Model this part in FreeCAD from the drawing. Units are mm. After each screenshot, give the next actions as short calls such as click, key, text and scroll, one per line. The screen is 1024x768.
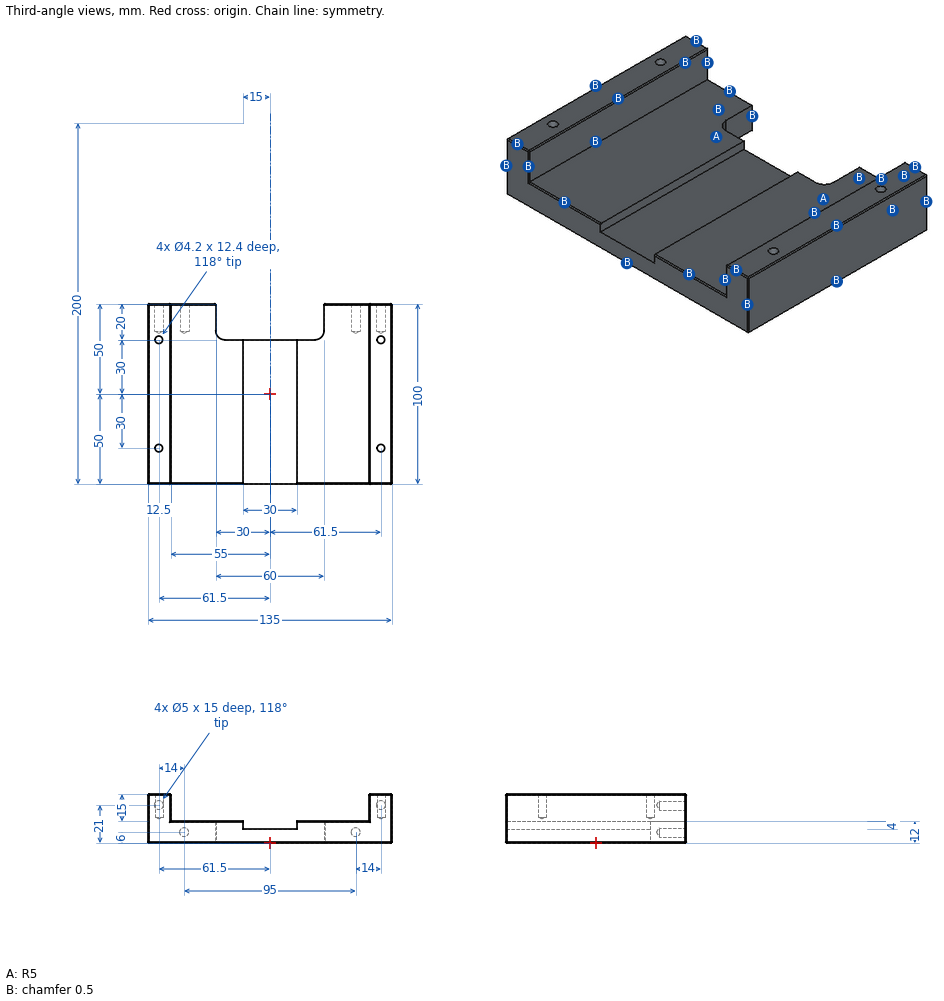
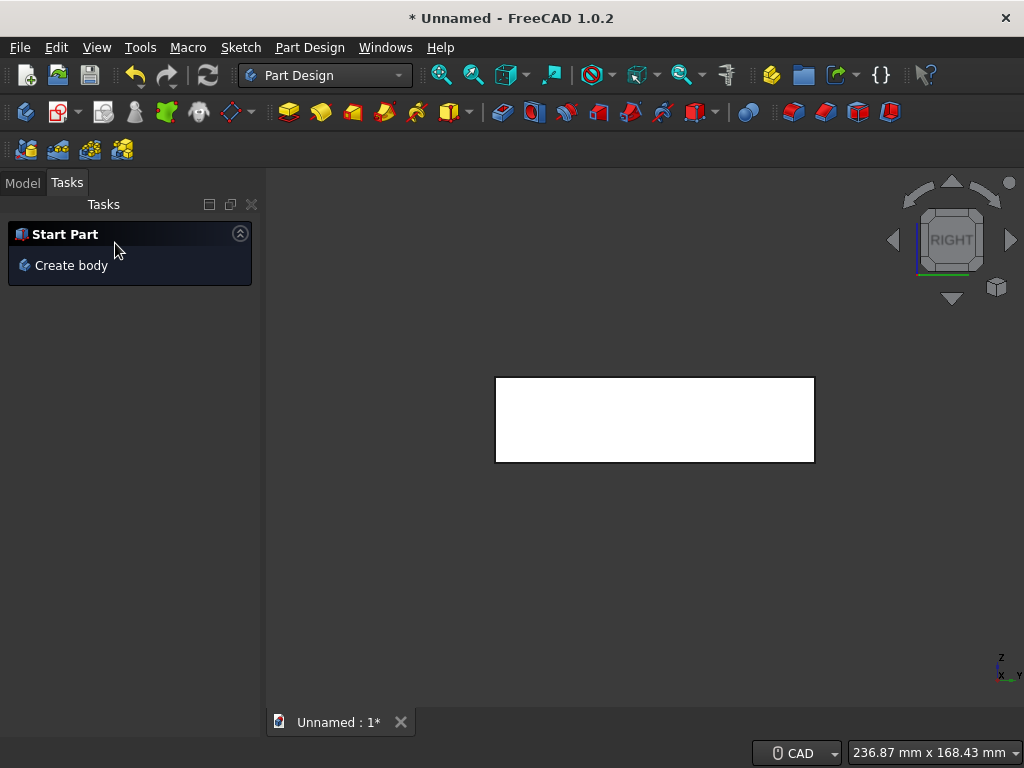
click(442, 76)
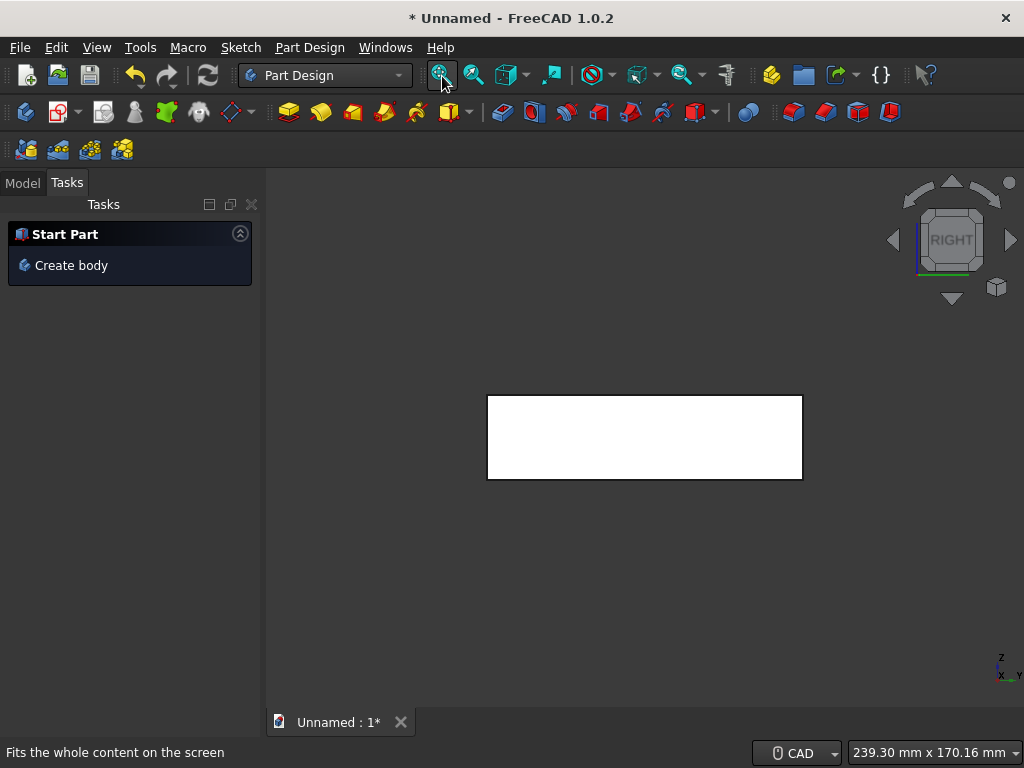
key(5)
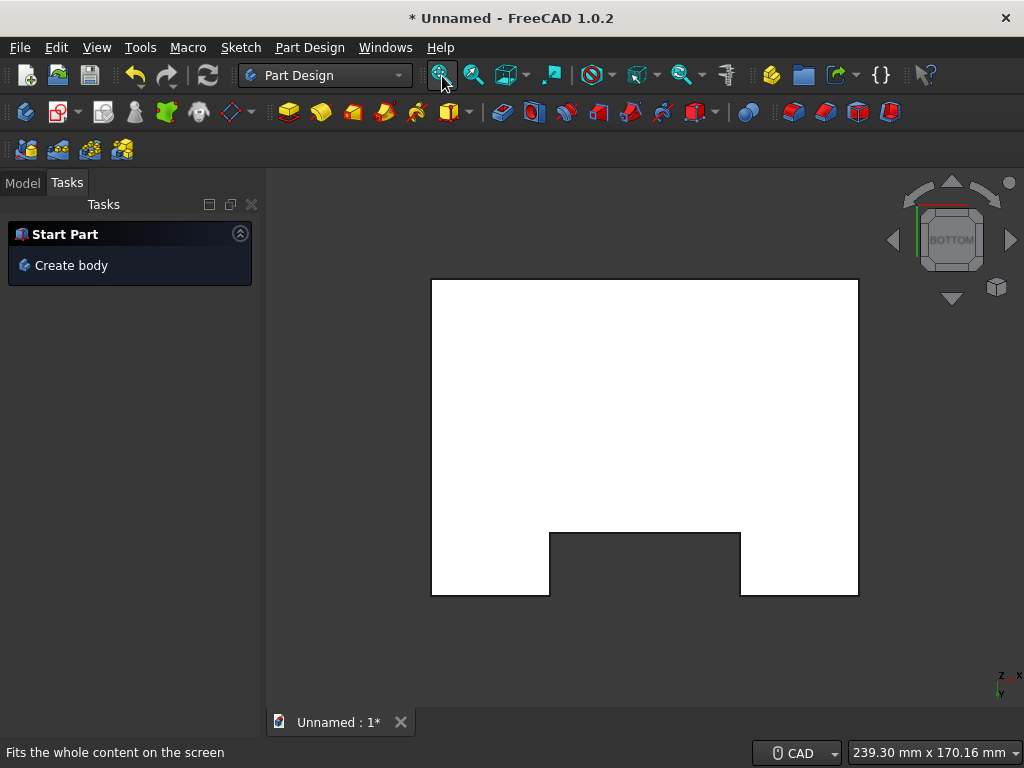
key(4)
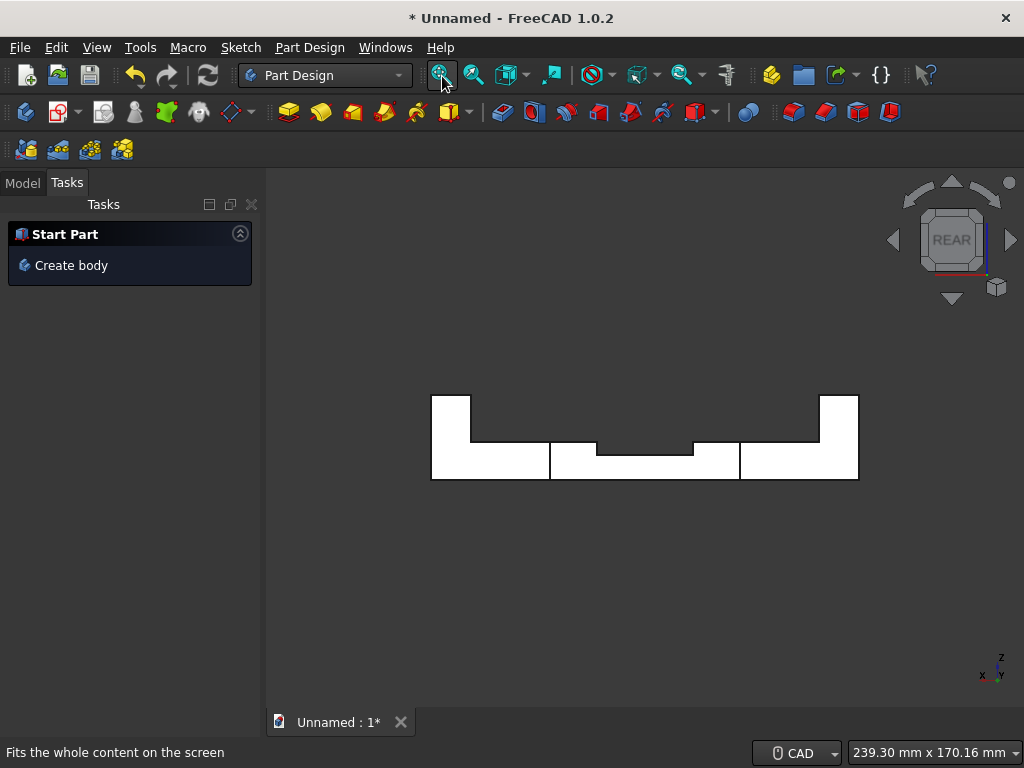
key(6)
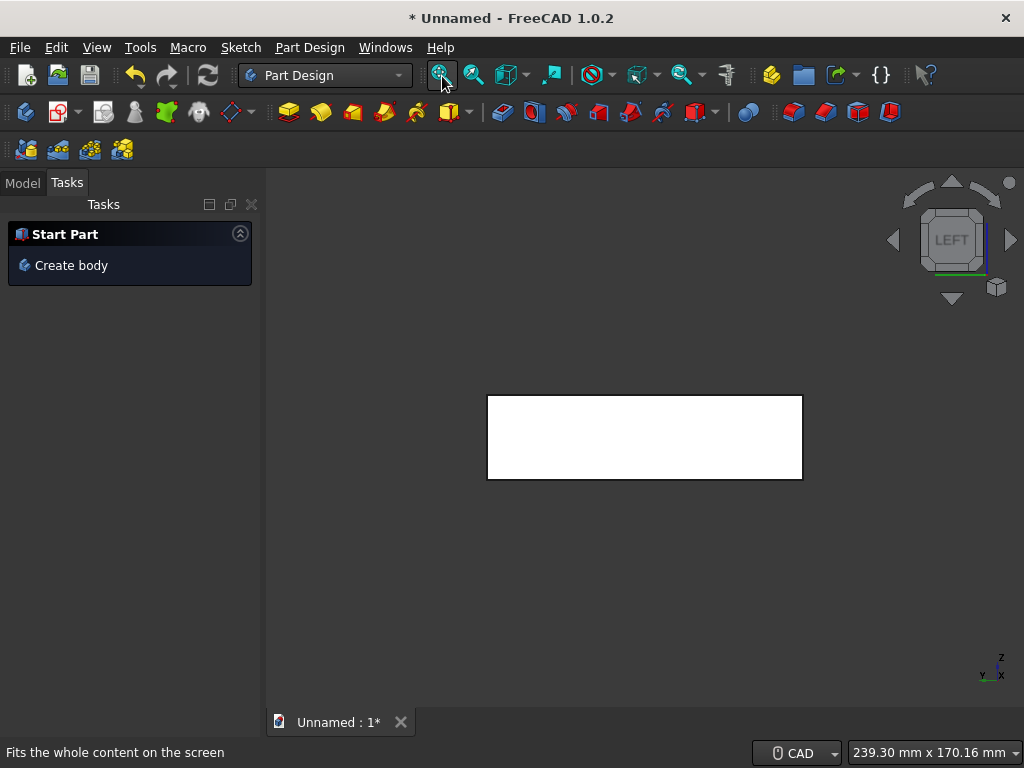
click(442, 76)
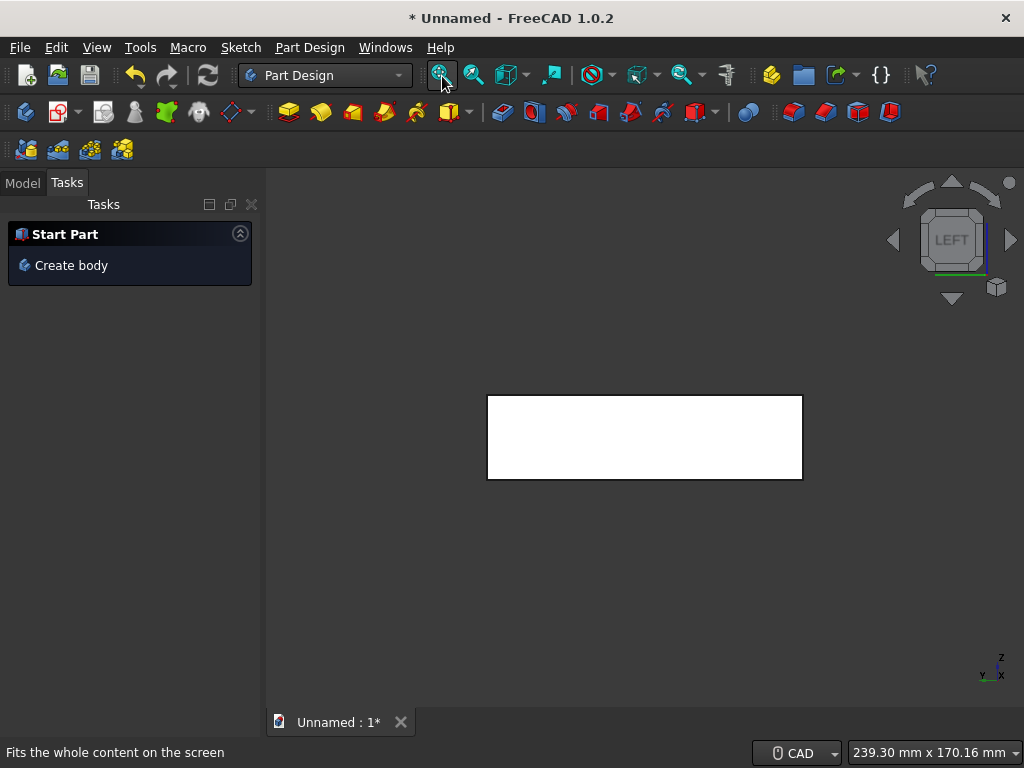
key(v)
key(3)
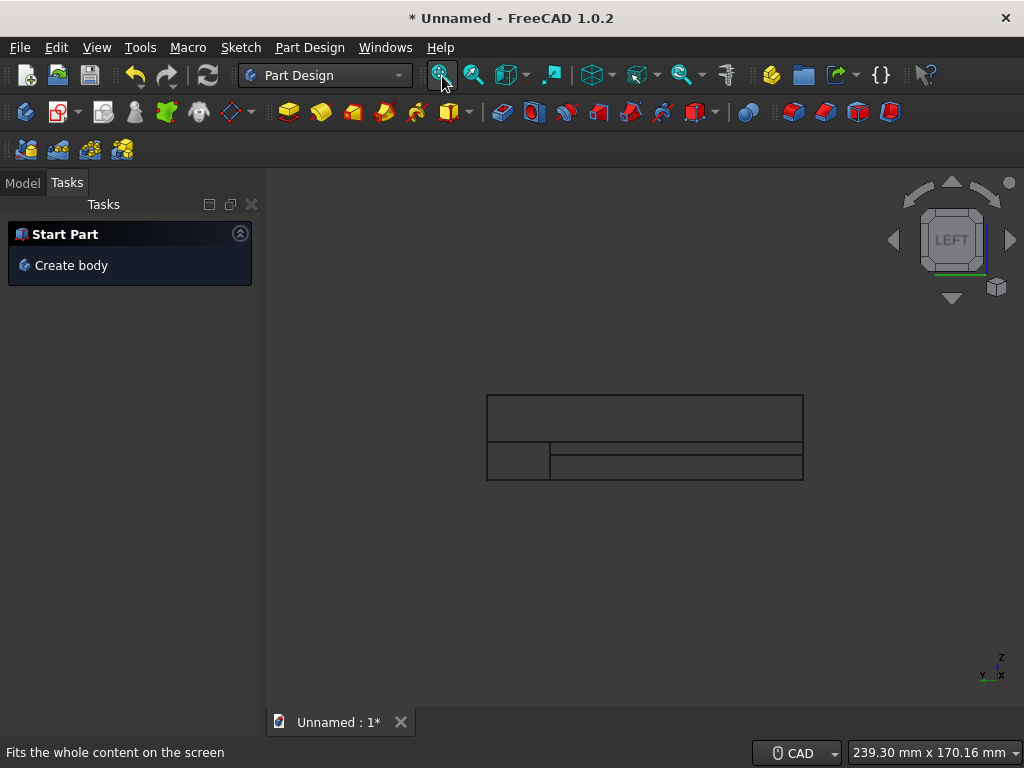
key(0)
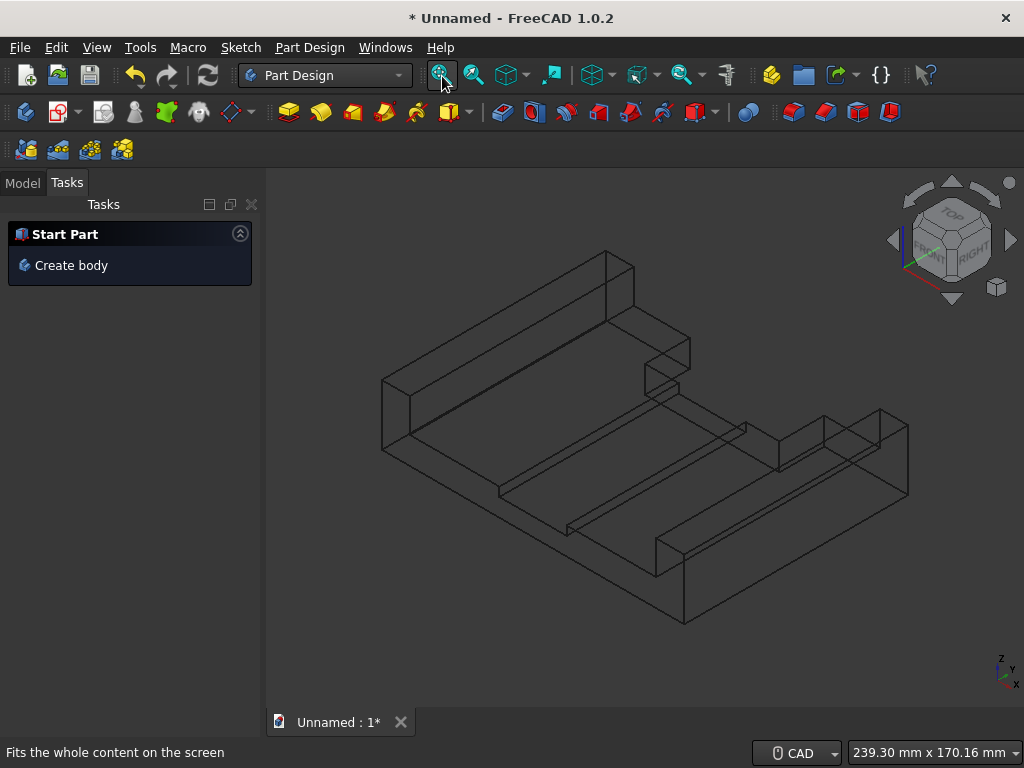
click(779, 456)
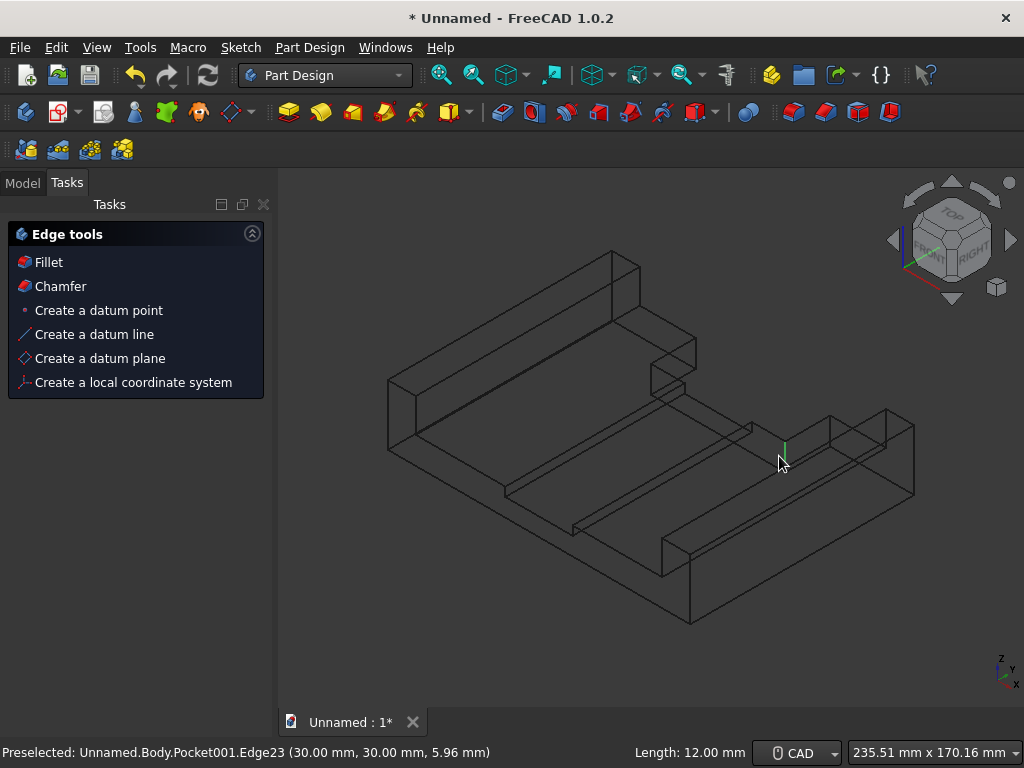
click(651, 378, ctrl)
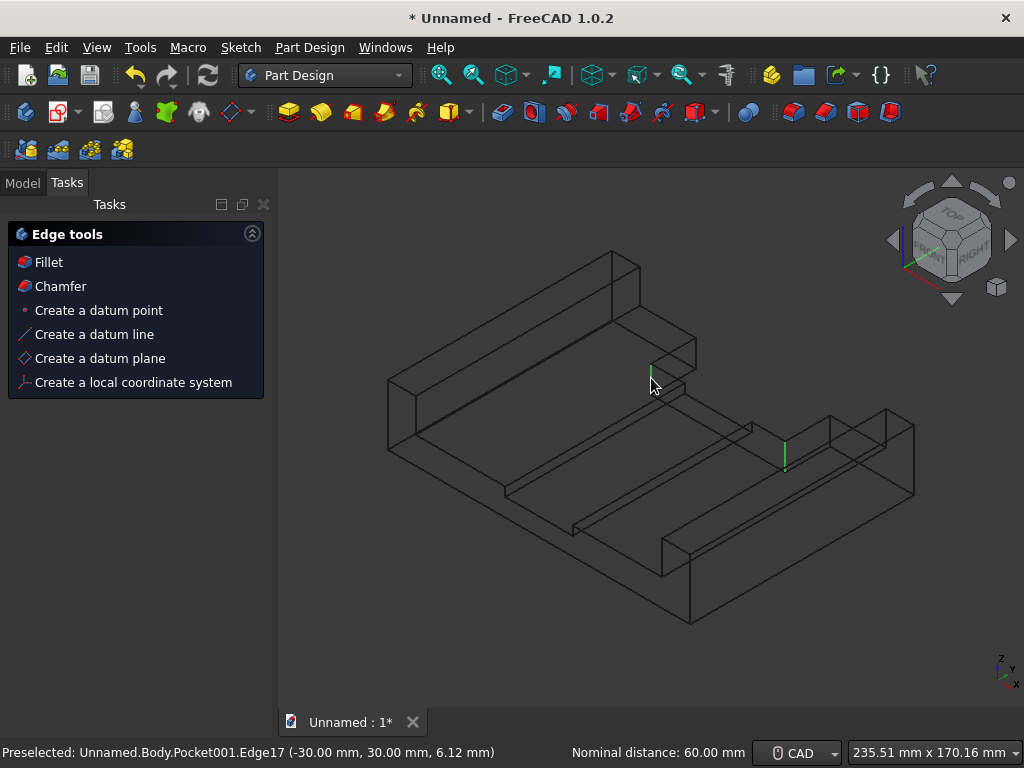
key(v)
key(1)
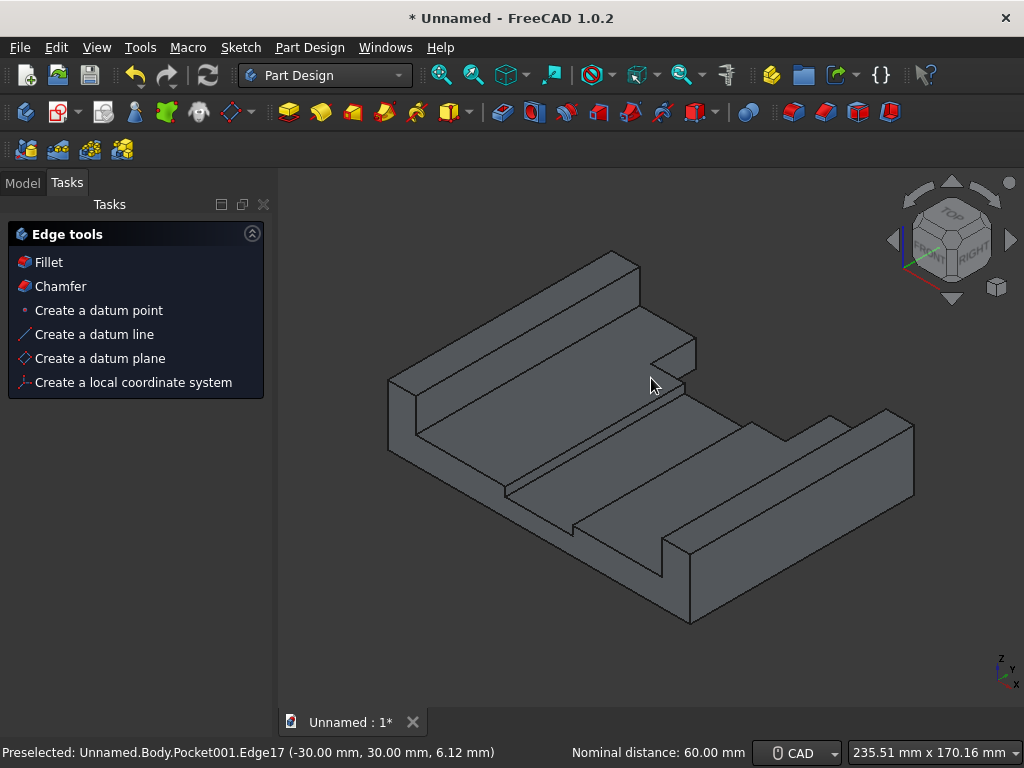
click(794, 112)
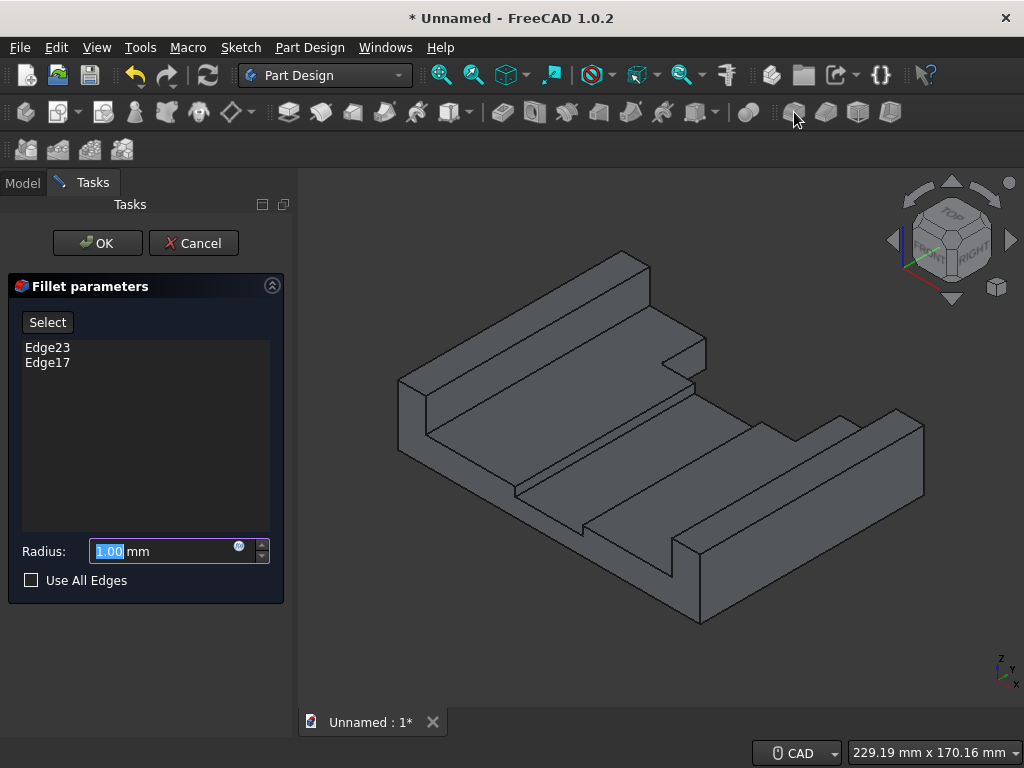
text(5)
key(Tab)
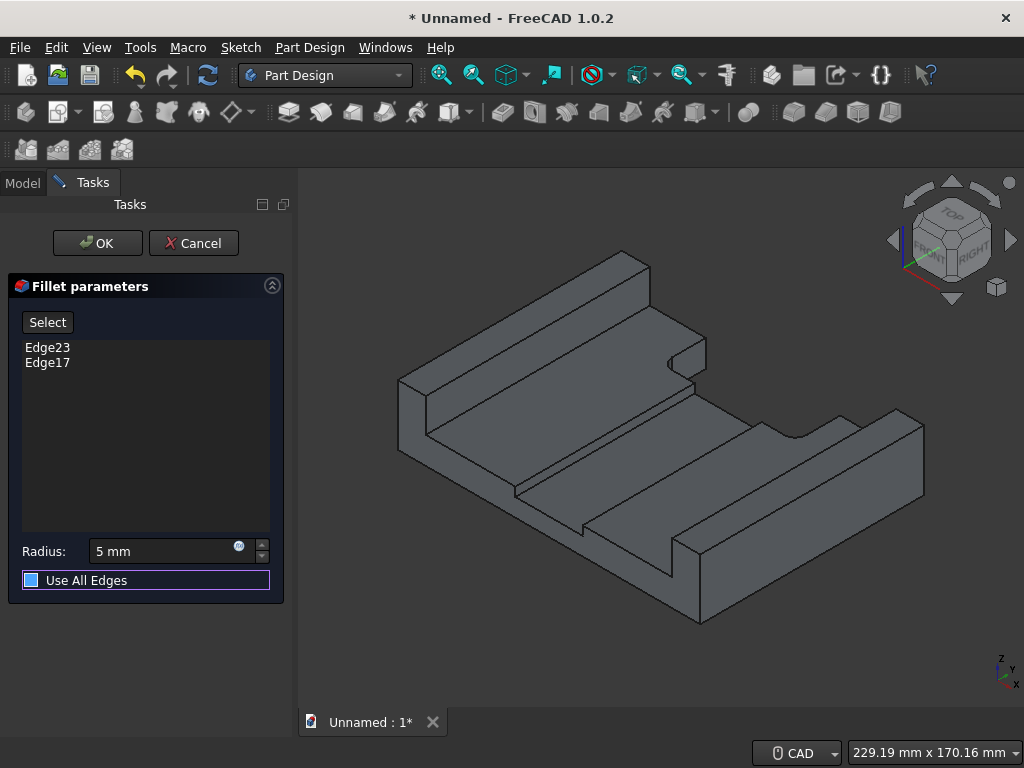
click(98, 243)